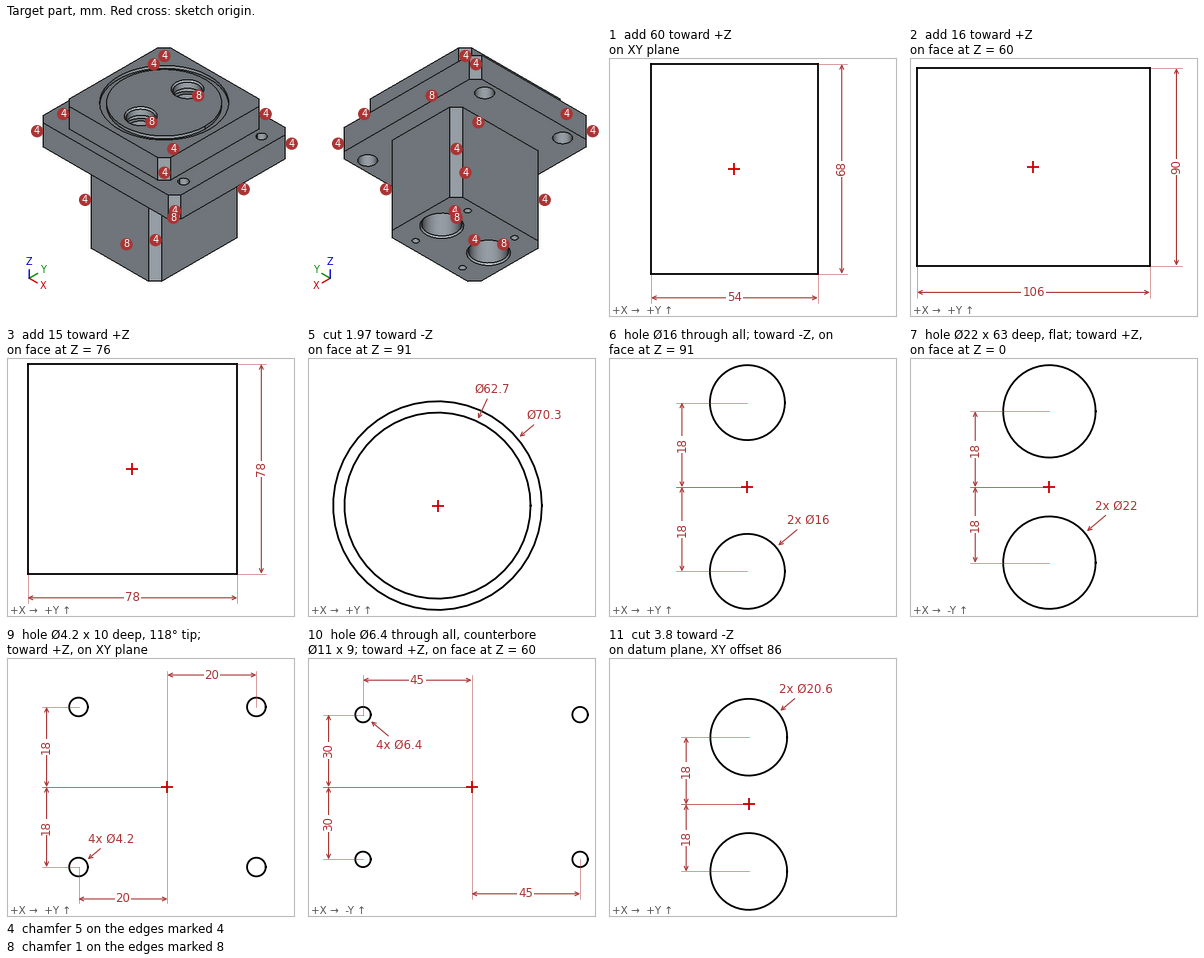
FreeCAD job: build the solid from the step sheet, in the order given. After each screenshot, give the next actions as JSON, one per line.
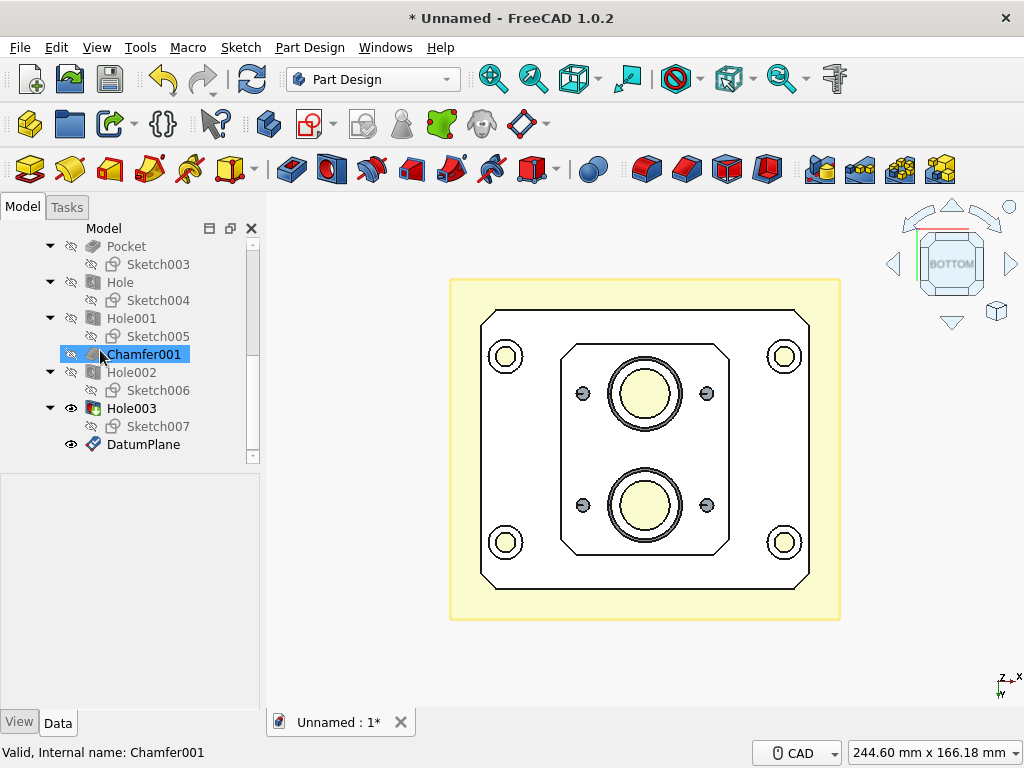
{"action": "left_click", "coordinate": [116, 444]}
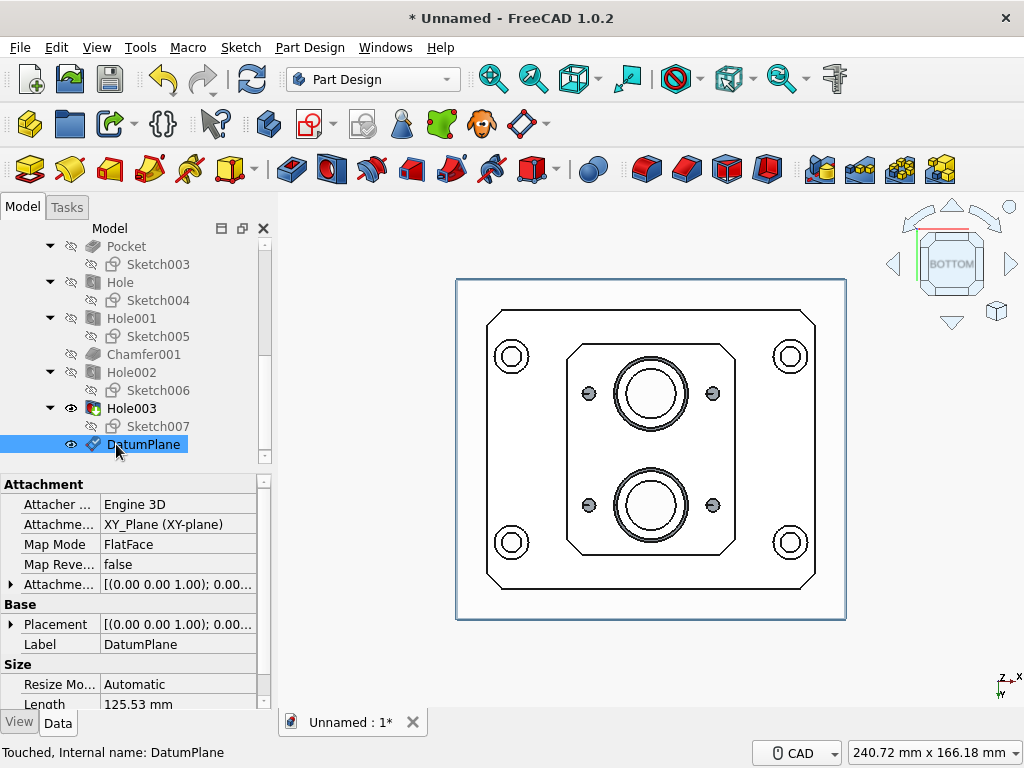
{"action": "left_click", "coordinate": [310, 124]}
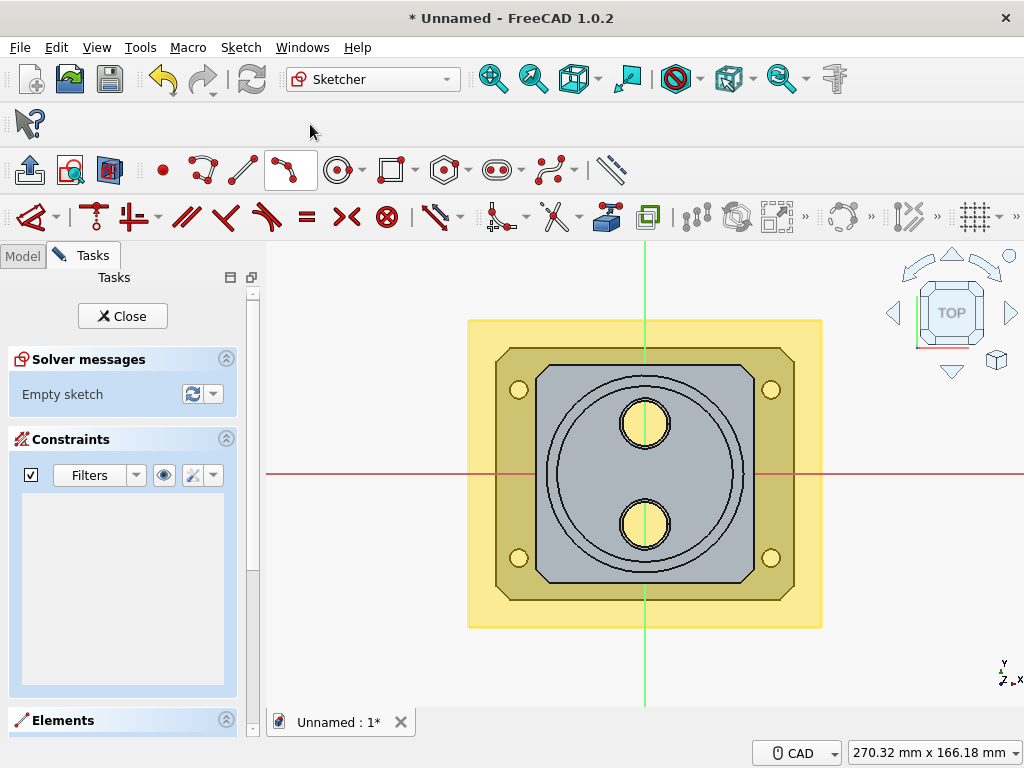
{"action": "key", "text": "q s"}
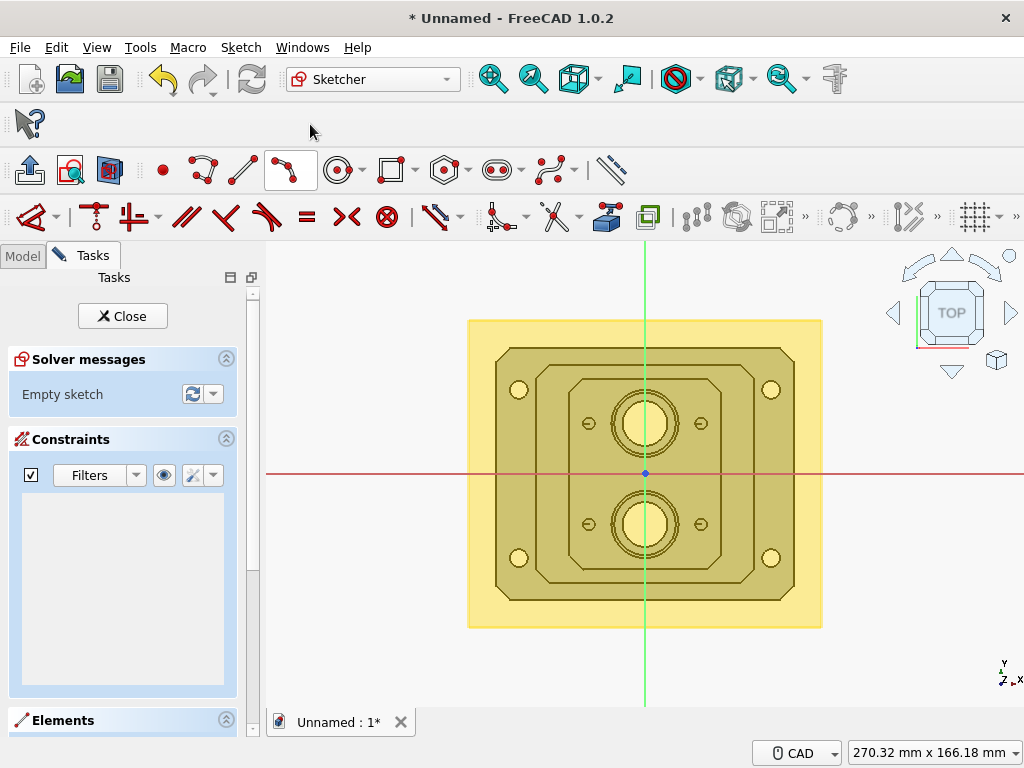
{"action": "scroll", "coordinate": [728, 474], "scroll_direction": "up", "scroll_amount": 3}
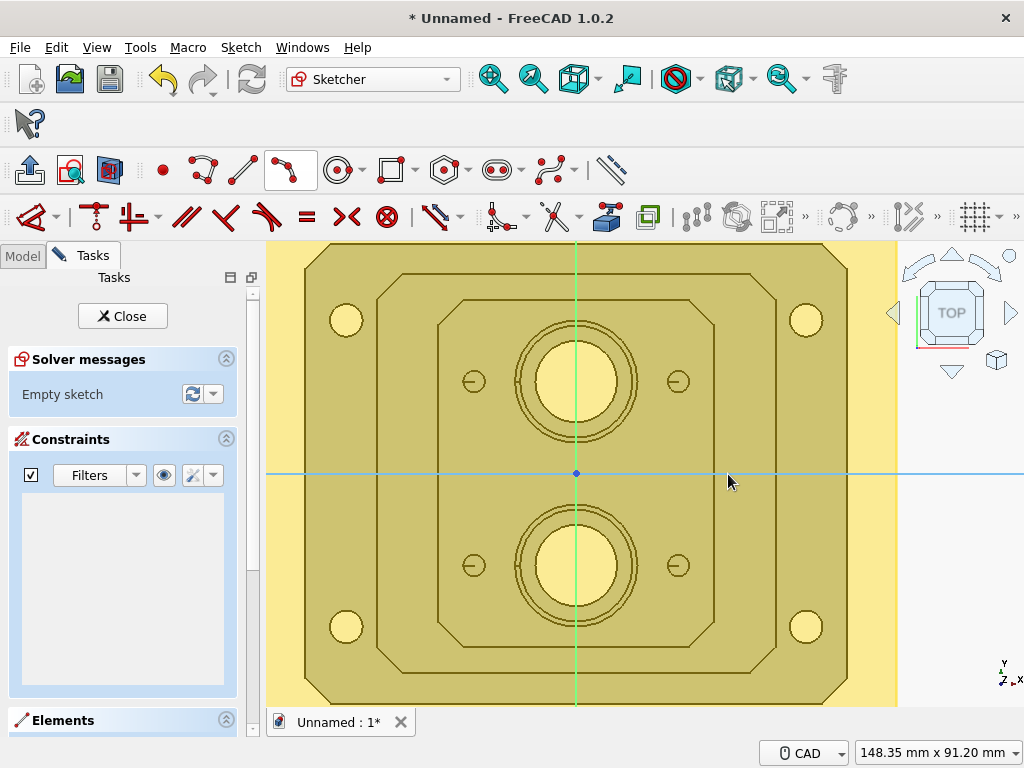
{"action": "left_click", "coordinate": [338, 170]}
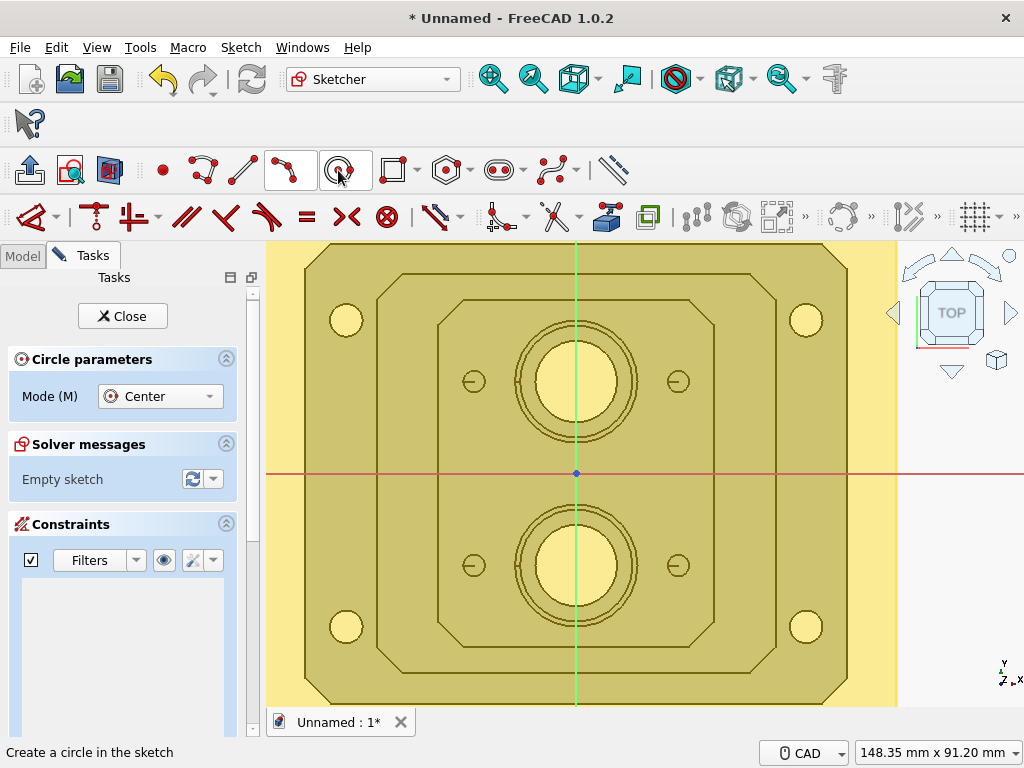
{"action": "left_click", "coordinate": [576, 382]}
{"action": "mouse_move", "coordinate": [613, 344]}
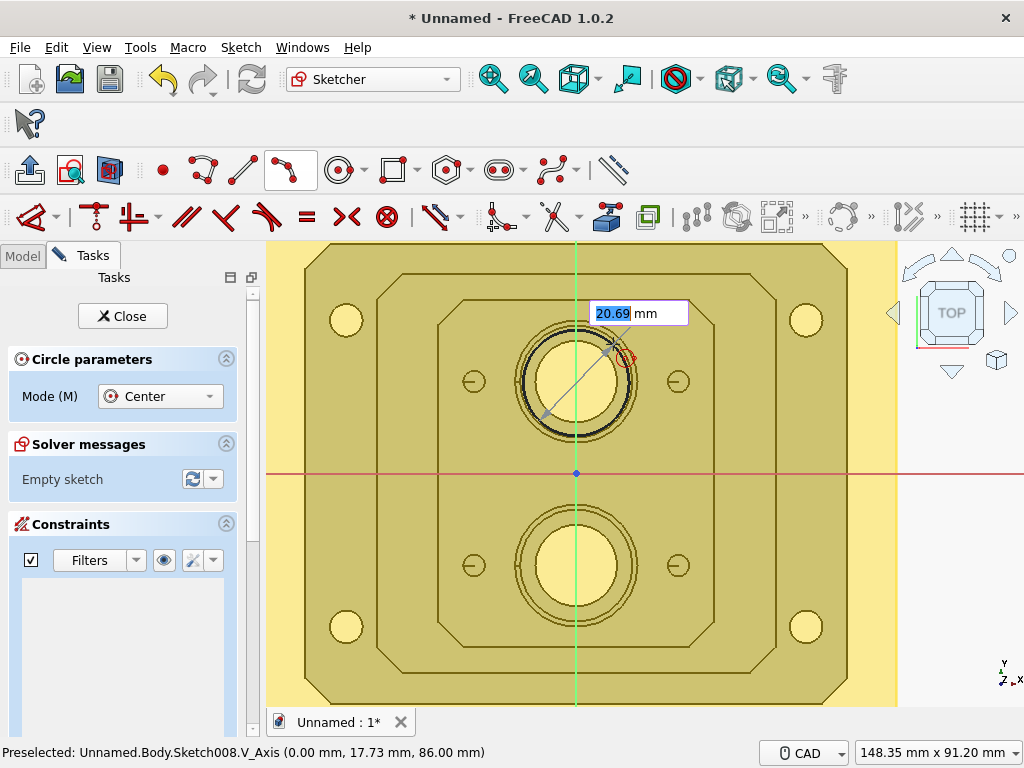
{"action": "type", "text": "20.6"}
{"action": "key", "text": "Return"}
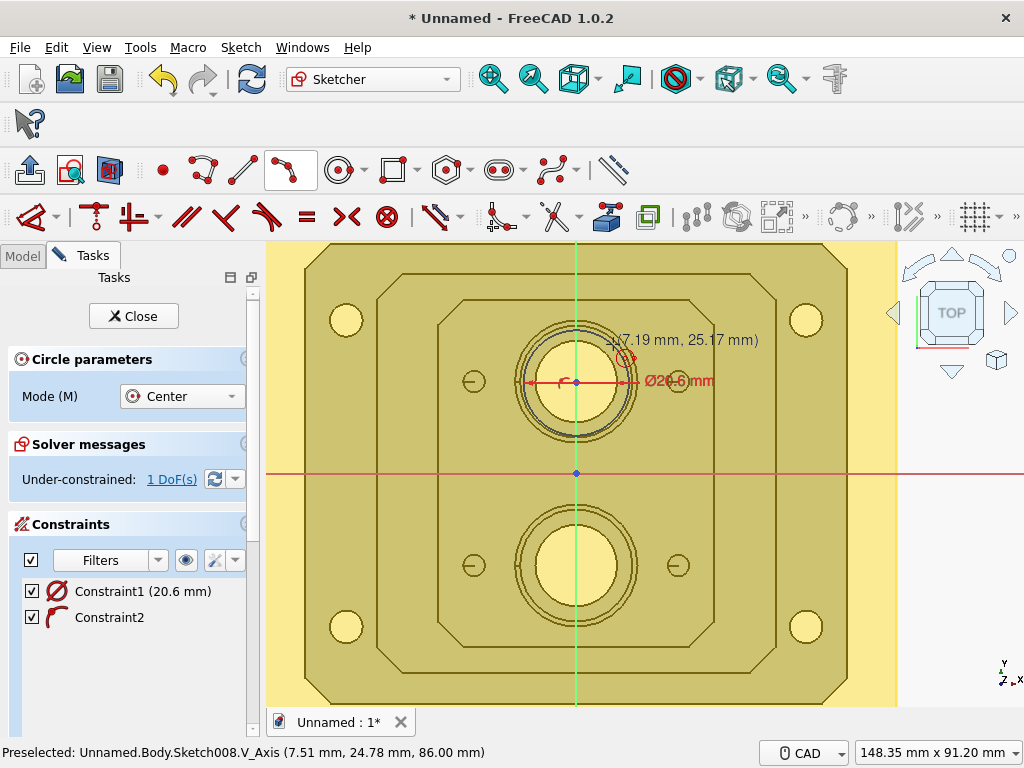
{"action": "left_click", "coordinate": [576, 566]}
{"action": "mouse_move", "coordinate": [613, 528]}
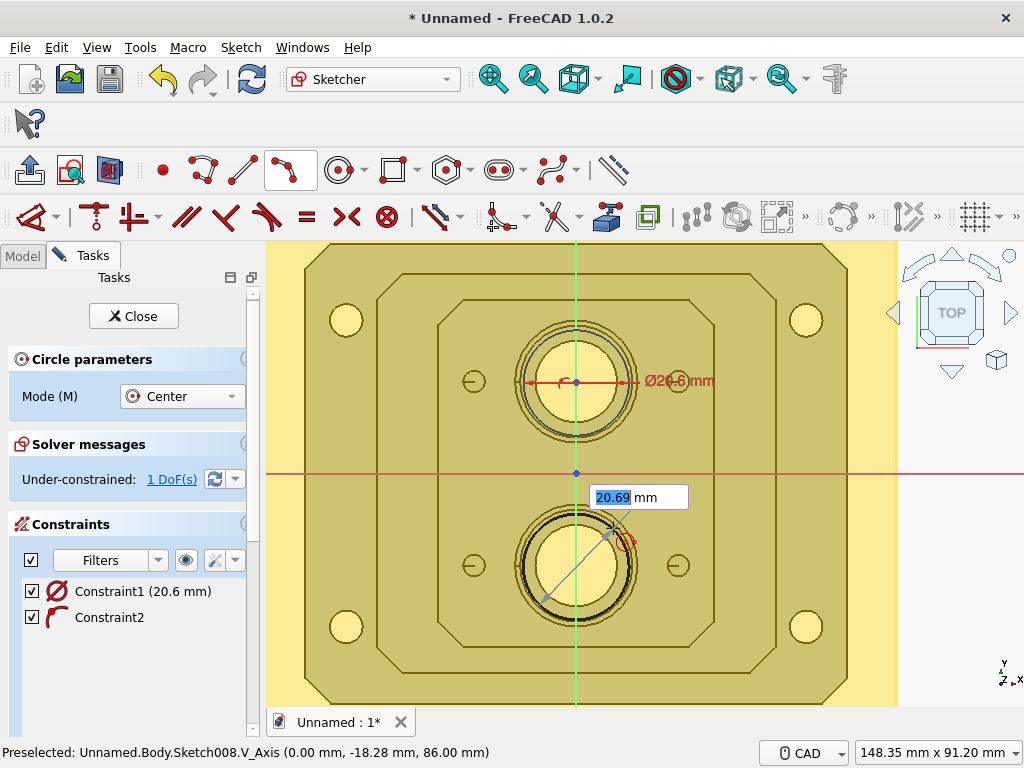
{"action": "type", "text": "20.6"}
{"action": "key", "text": "Return"}
{"action": "key", "text": "Escape"}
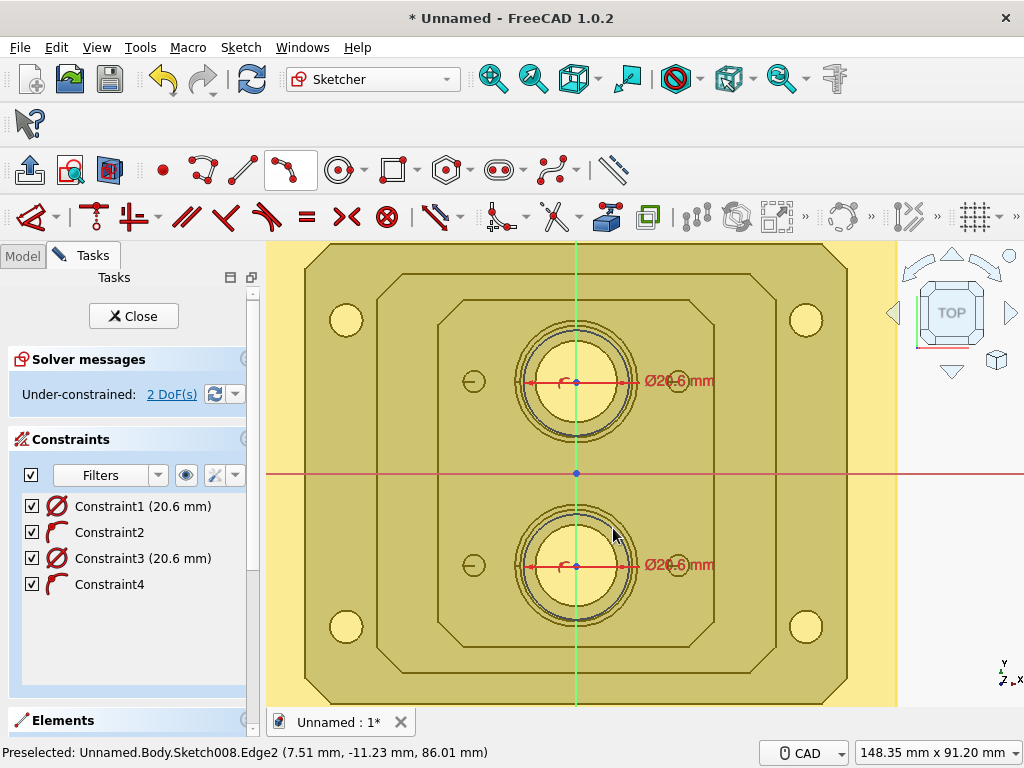
{"action": "key", "text": "d"}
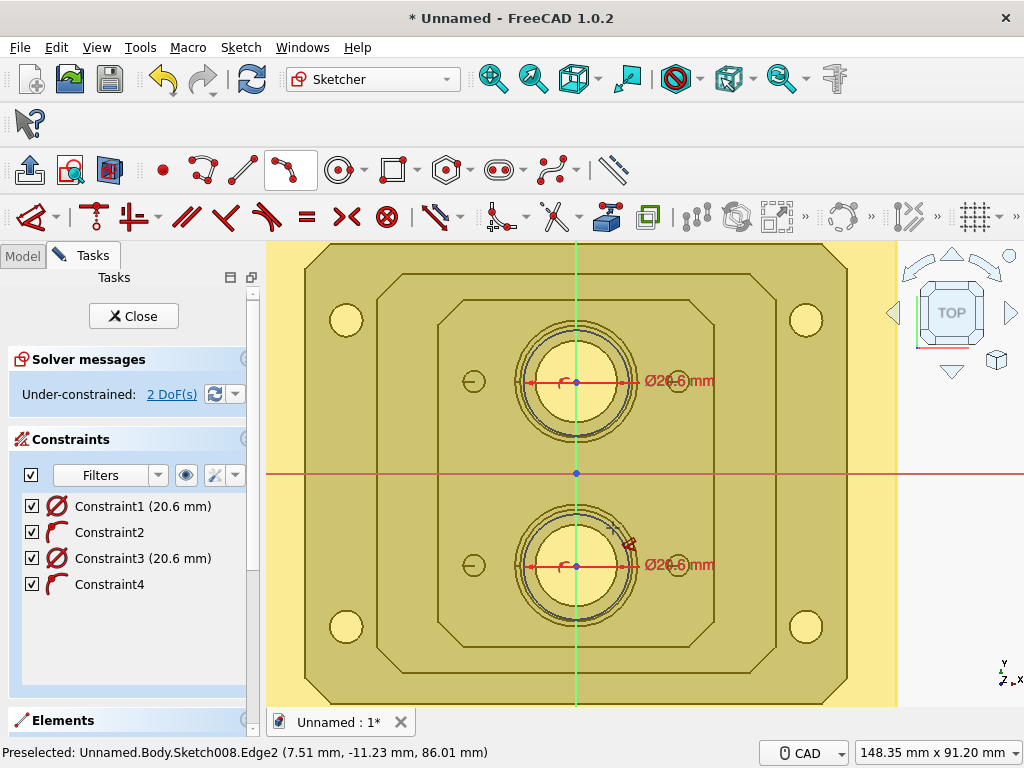
{"action": "left_click", "coordinate": [576, 383]}
{"action": "left_click", "coordinate": [610, 449]}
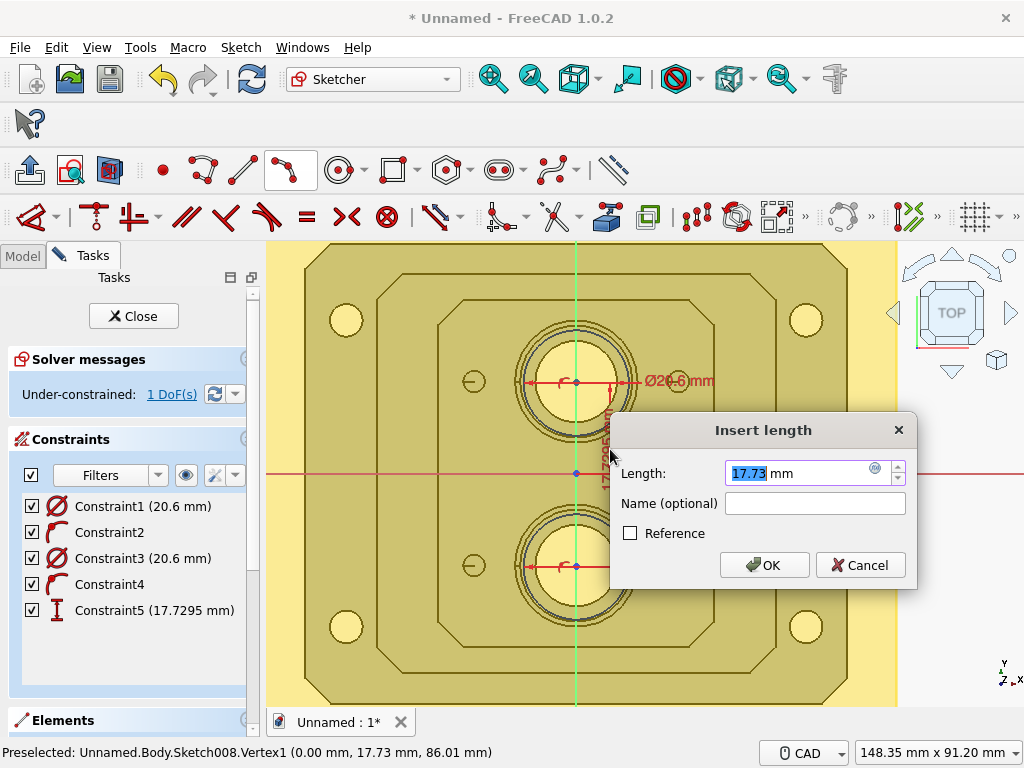
{"action": "type", "text": "18"}
{"action": "key", "text": "Return"}